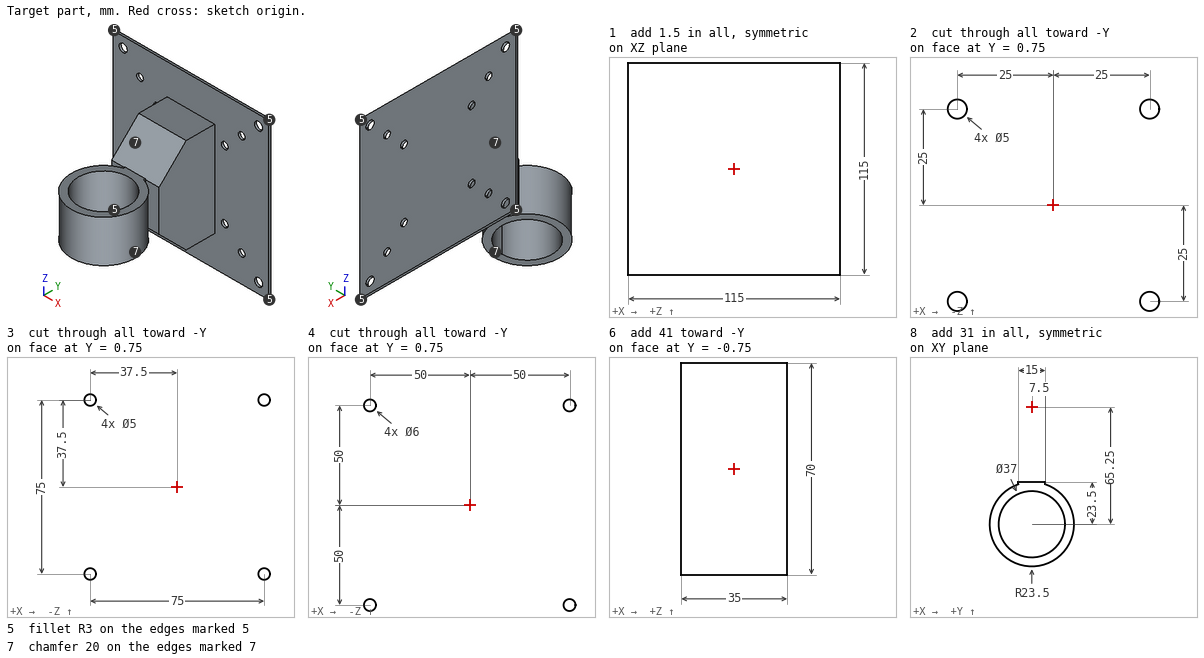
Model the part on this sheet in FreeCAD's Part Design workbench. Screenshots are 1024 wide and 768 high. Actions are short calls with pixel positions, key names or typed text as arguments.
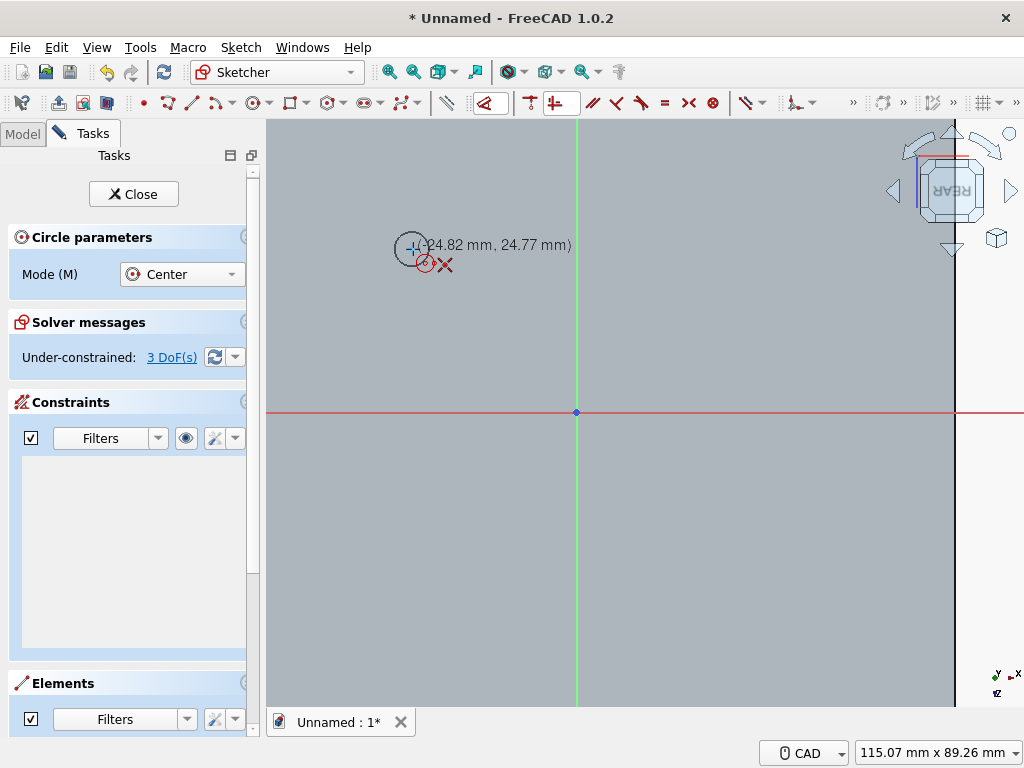
scroll(741, 248, up, 2)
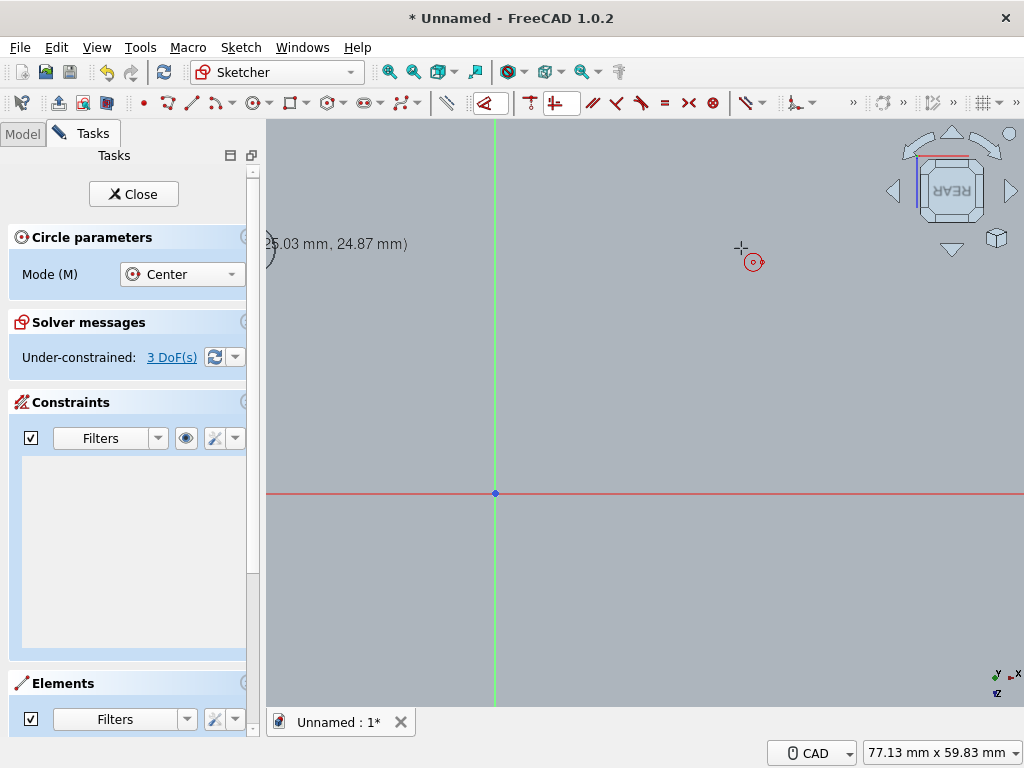
click(741, 248)
click(758, 231)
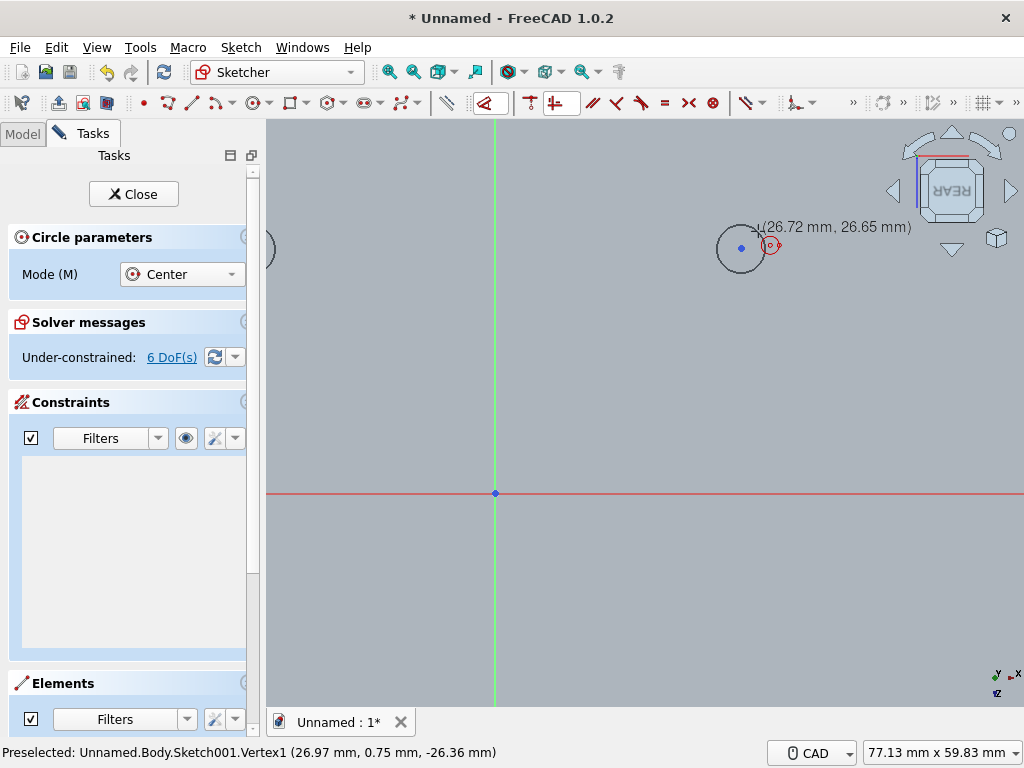
scroll(741, 248, down, 2)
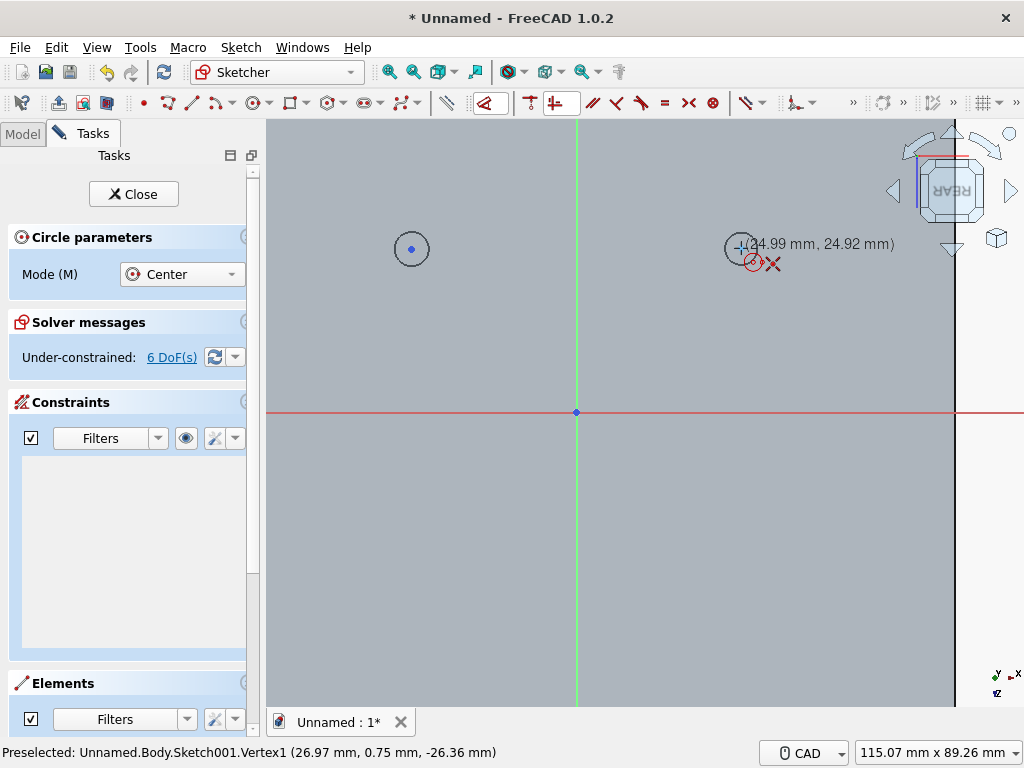
scroll(741, 578, up, 2)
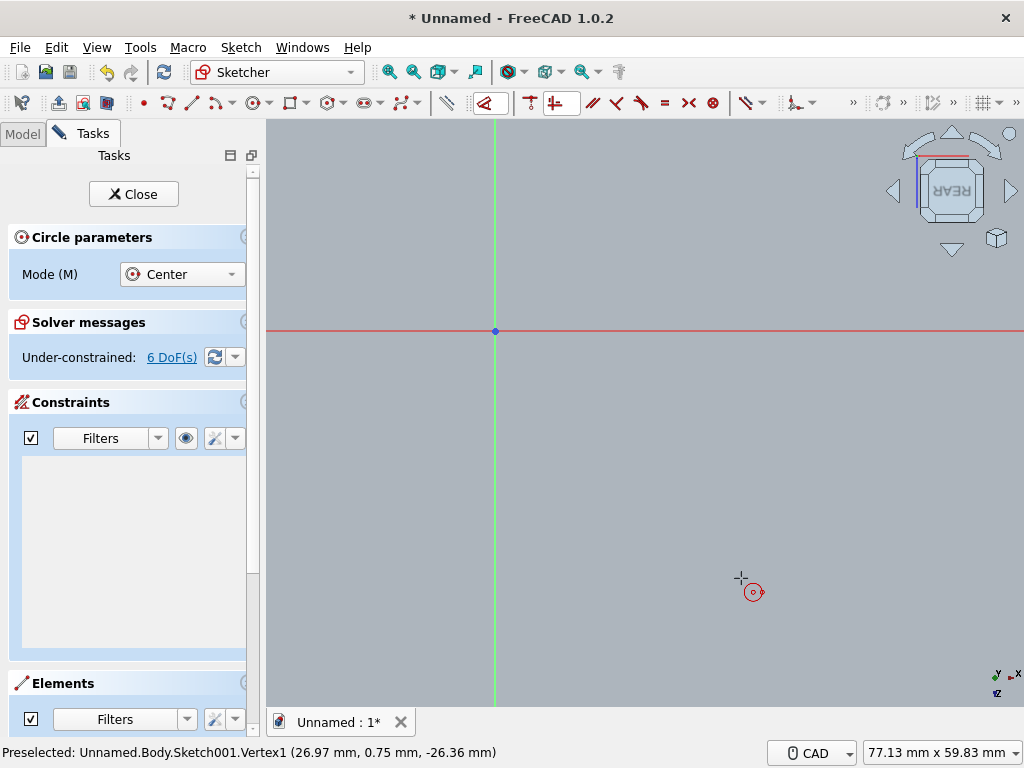
click(741, 577)
click(758, 560)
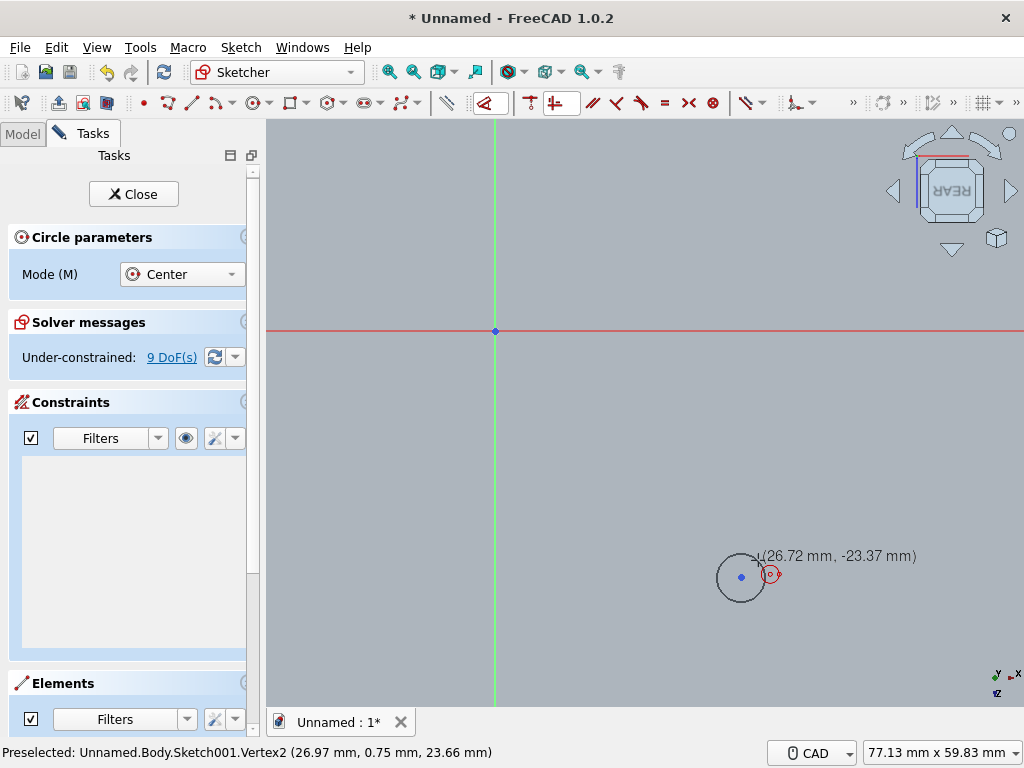
scroll(741, 579, down, 2)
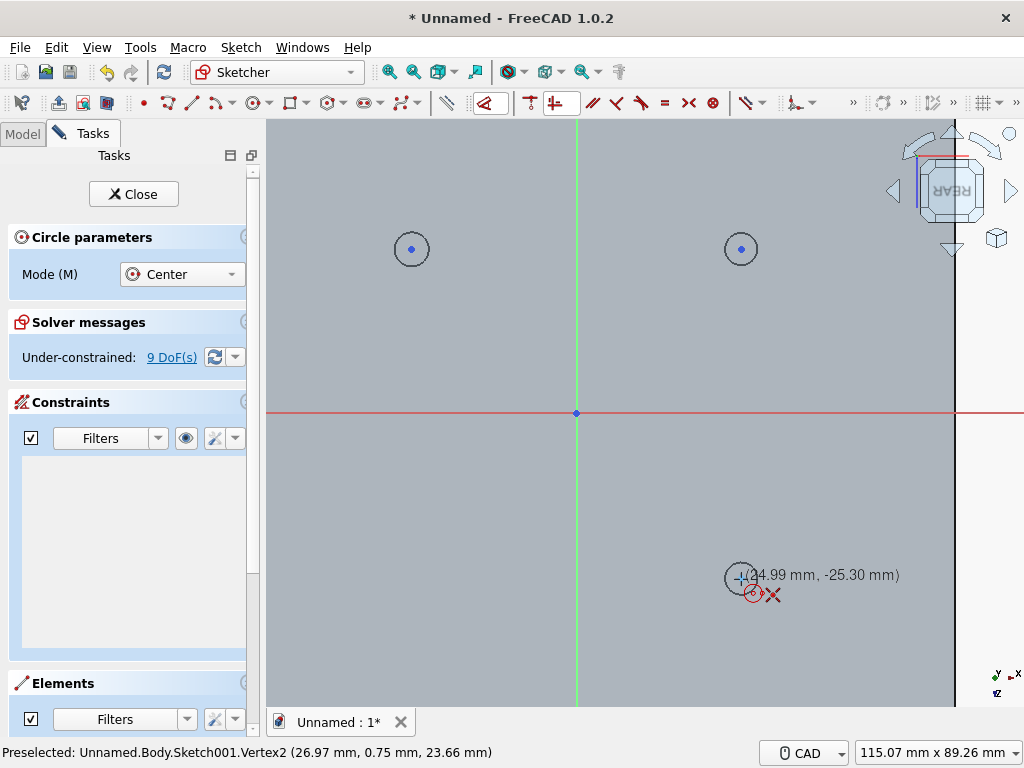
scroll(412, 578, up, 2)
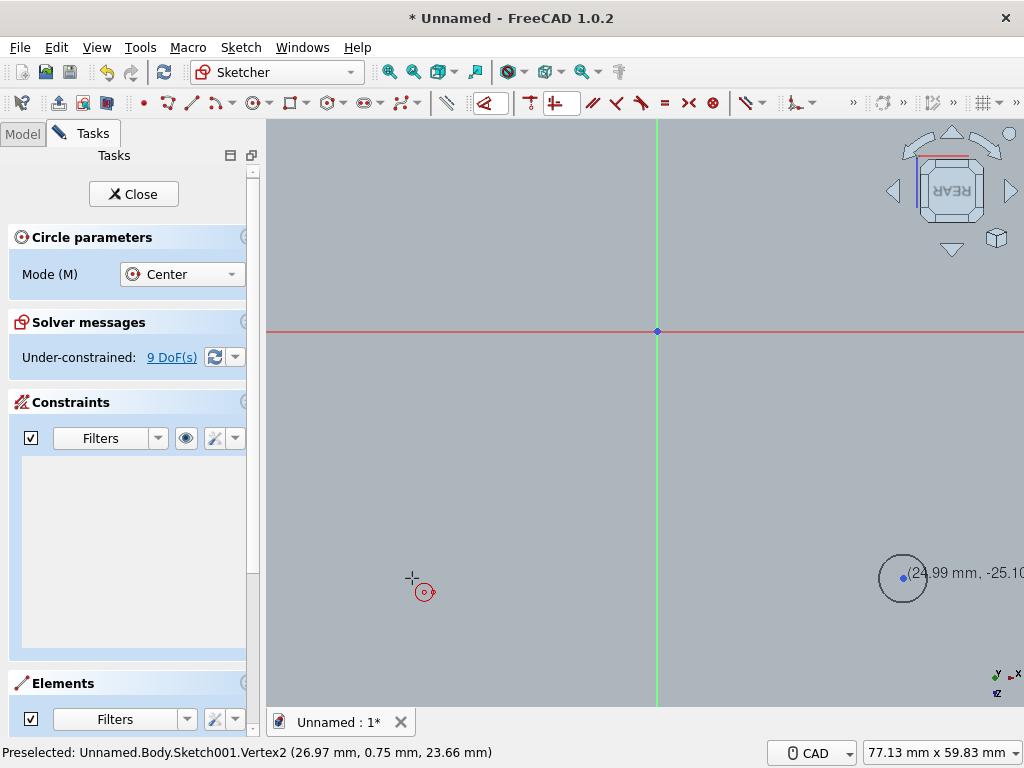
click(412, 578)
click(429, 560)
key(Escape)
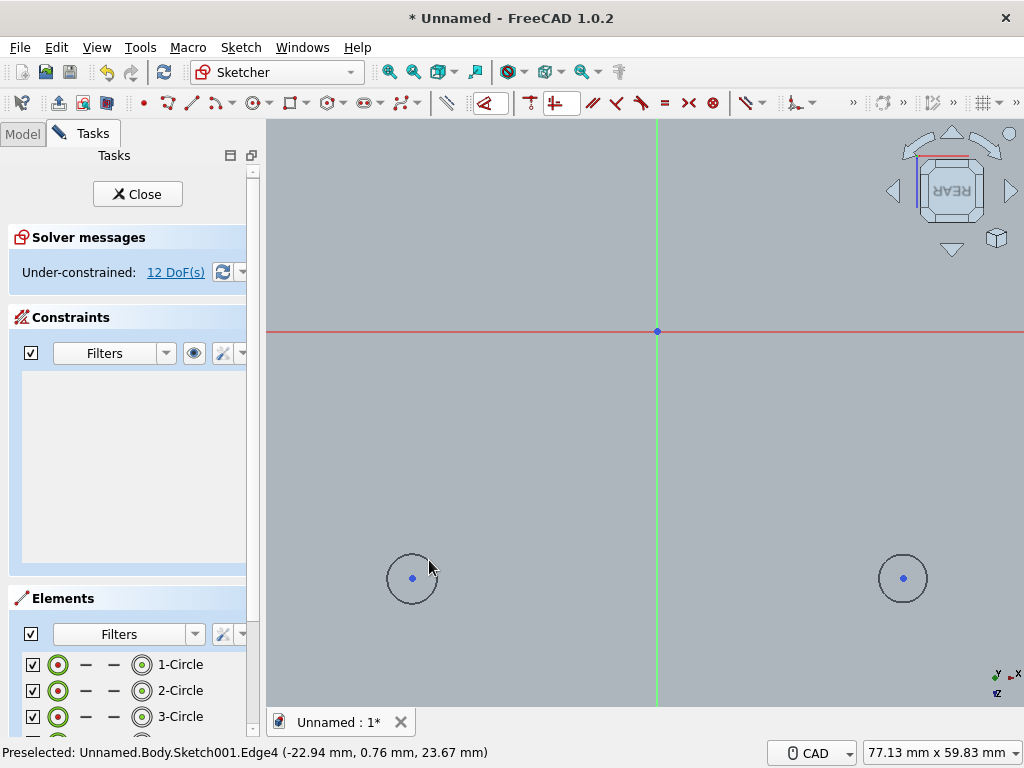
scroll(412, 578, down, 2)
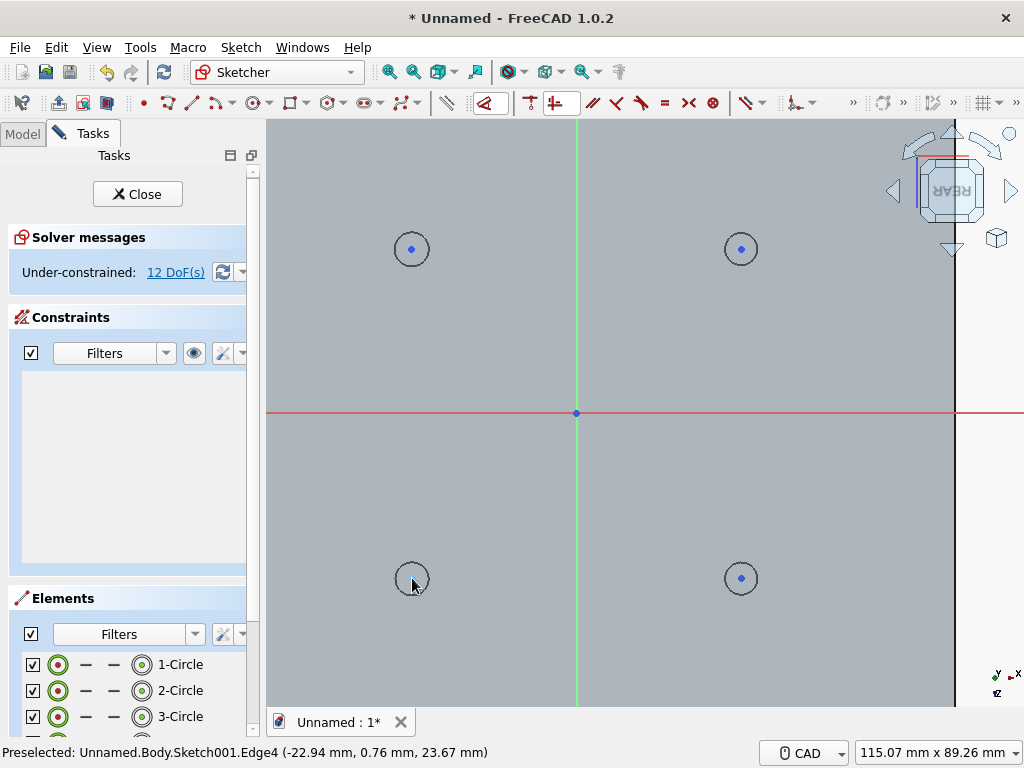
click(424, 237)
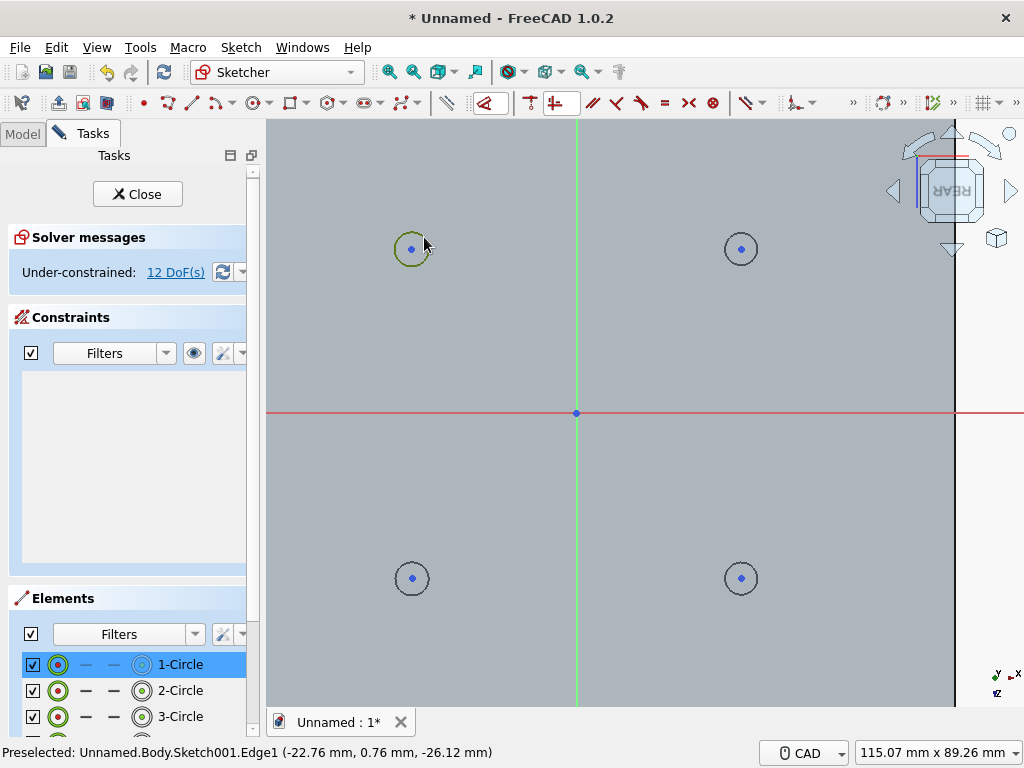
click(753, 238)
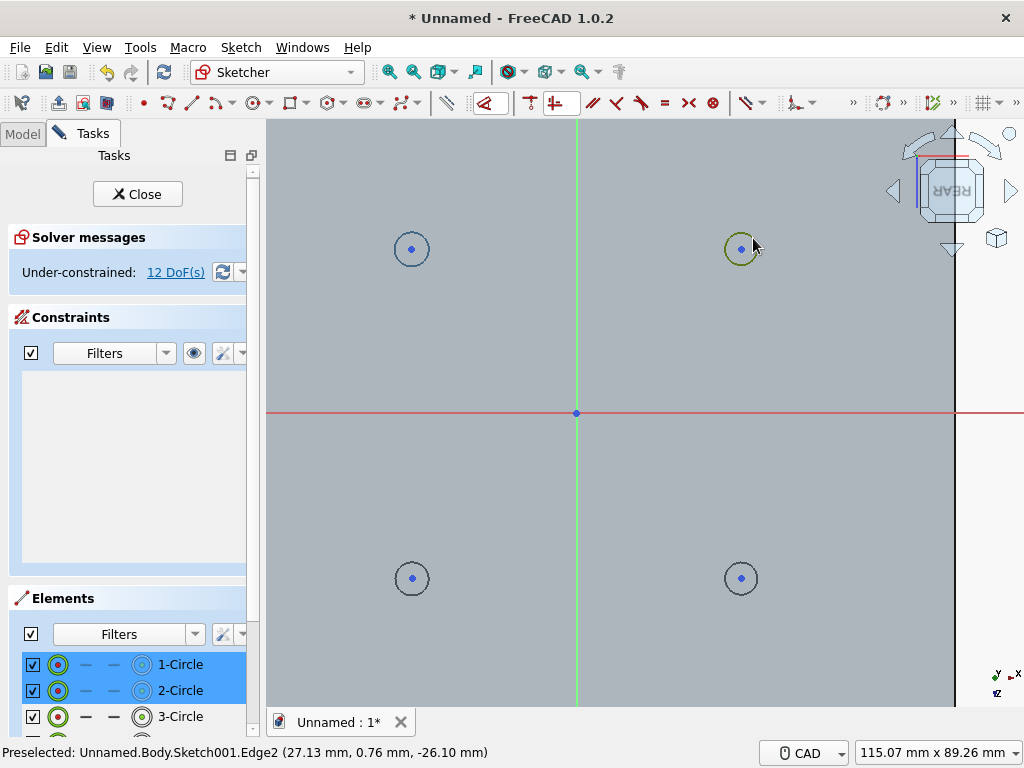
click(753, 567)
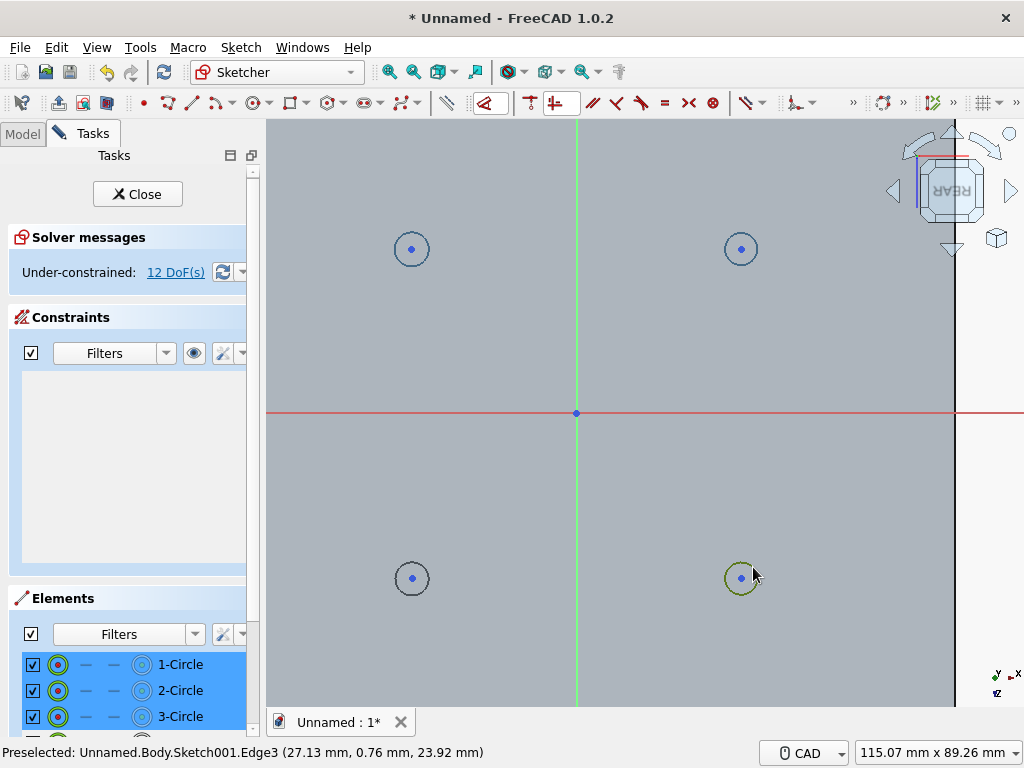
click(424, 567)